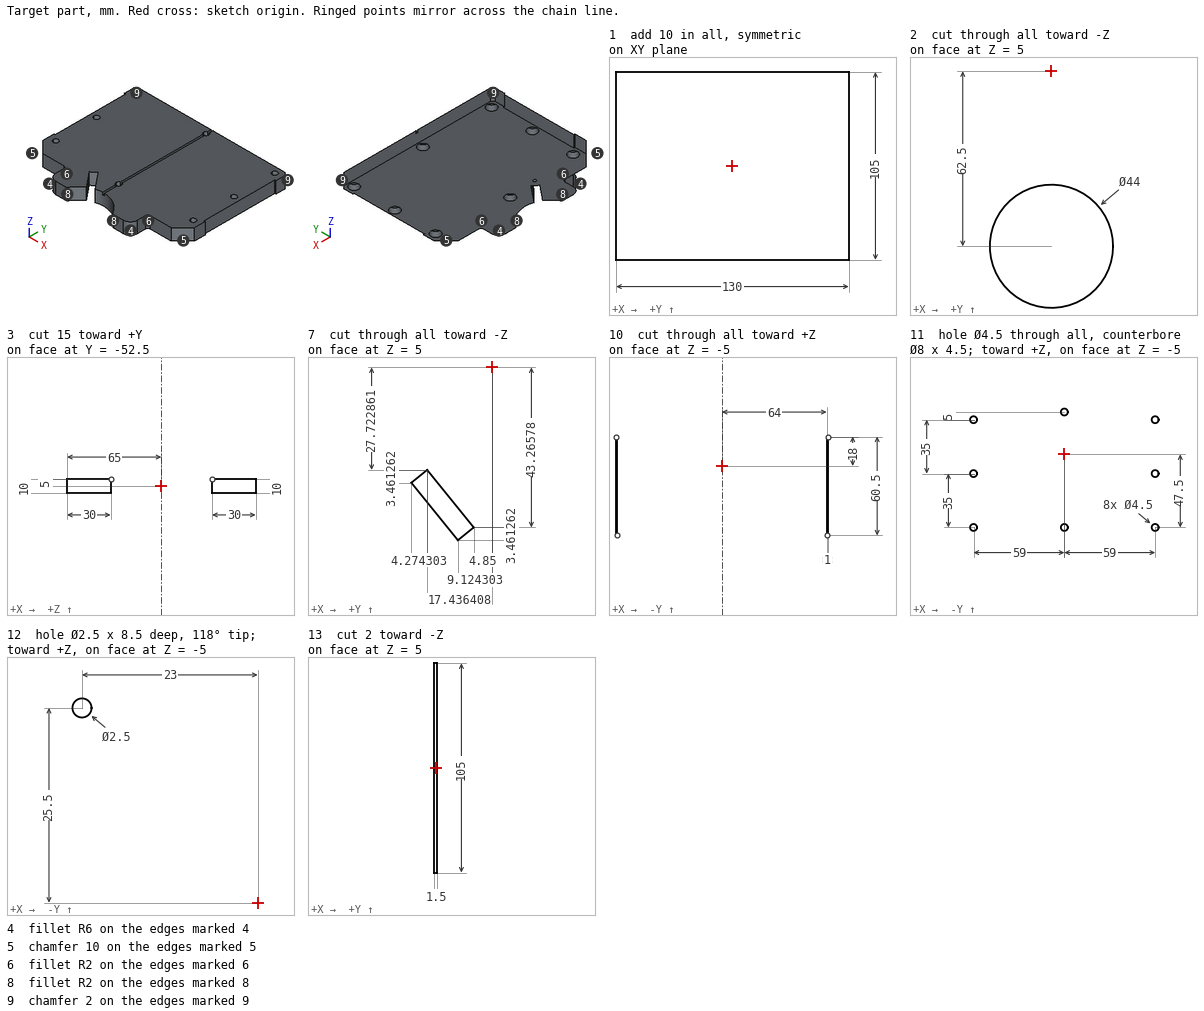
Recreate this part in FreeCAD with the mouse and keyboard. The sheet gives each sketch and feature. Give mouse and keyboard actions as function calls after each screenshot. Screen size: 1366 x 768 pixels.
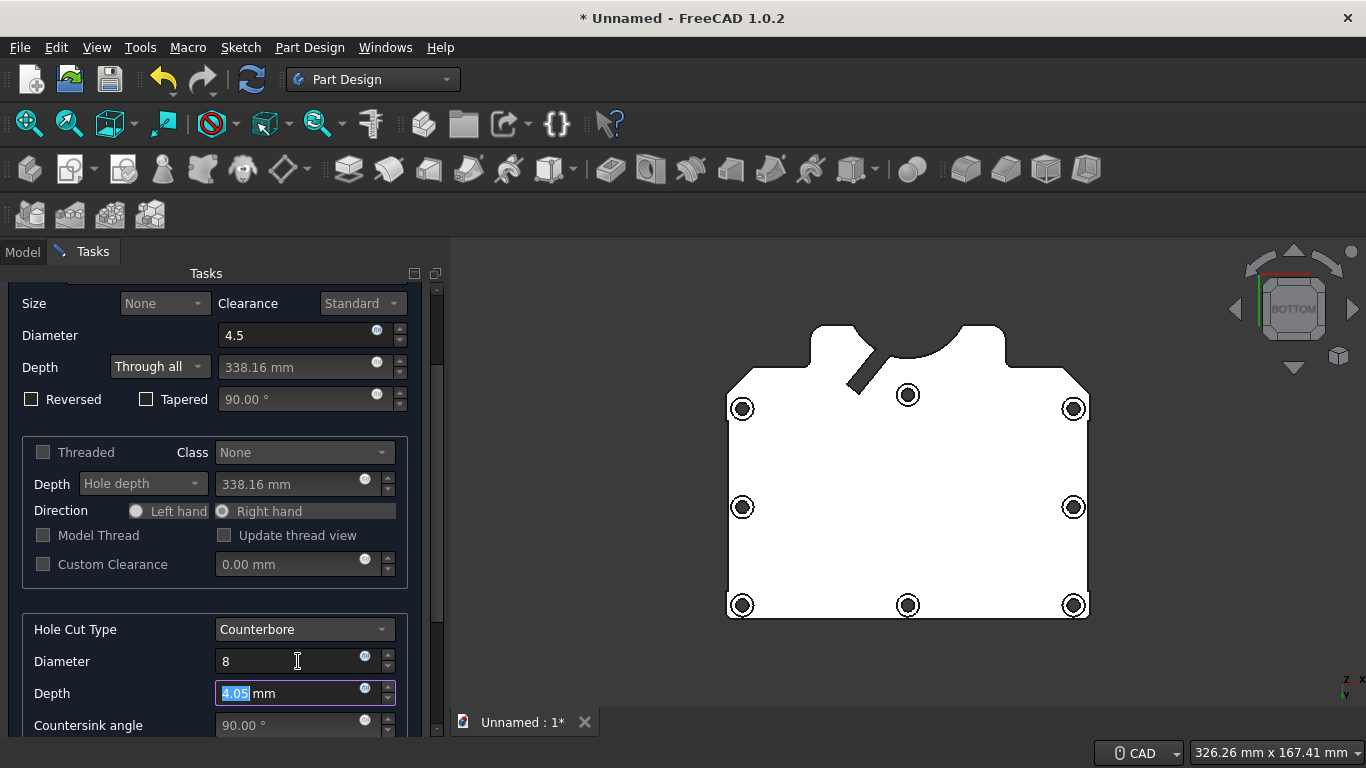
text(4.5)
key(Tab)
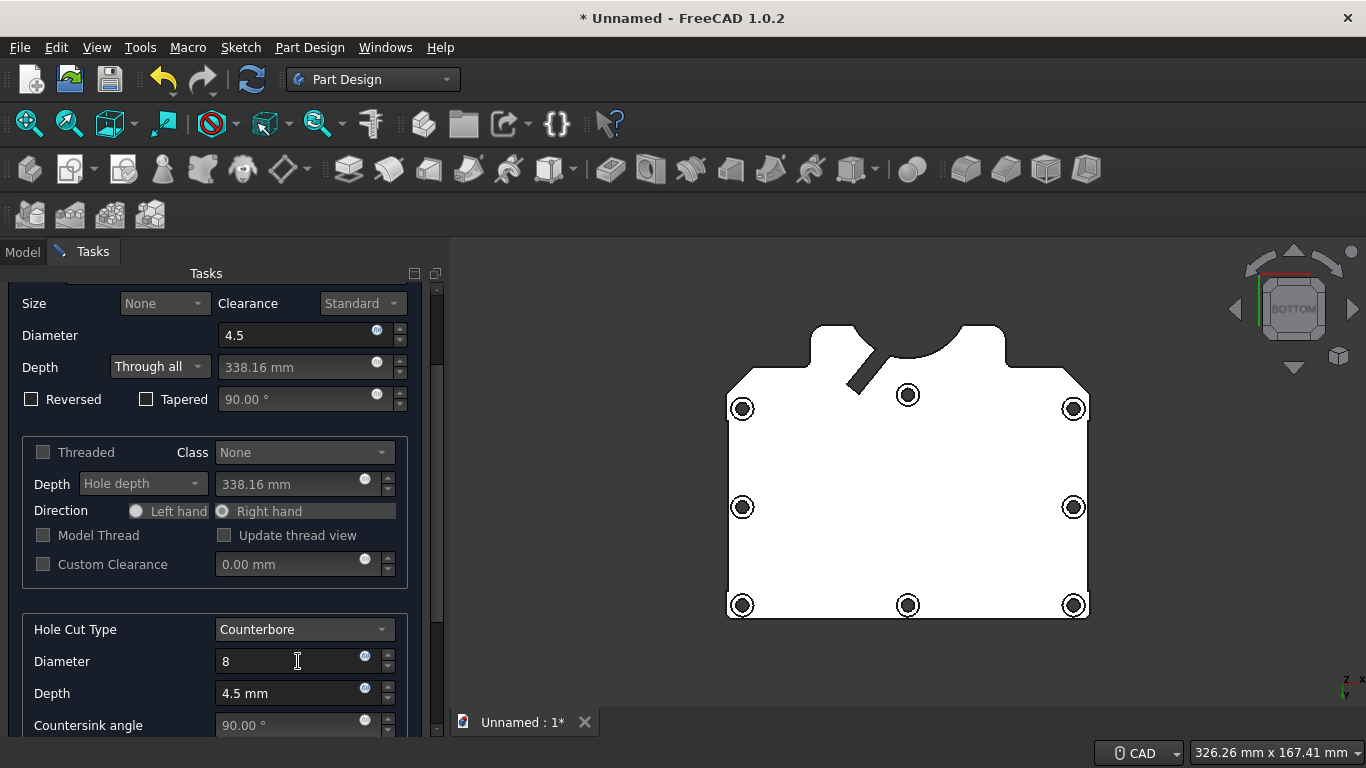
scroll(437, 510, up, 3)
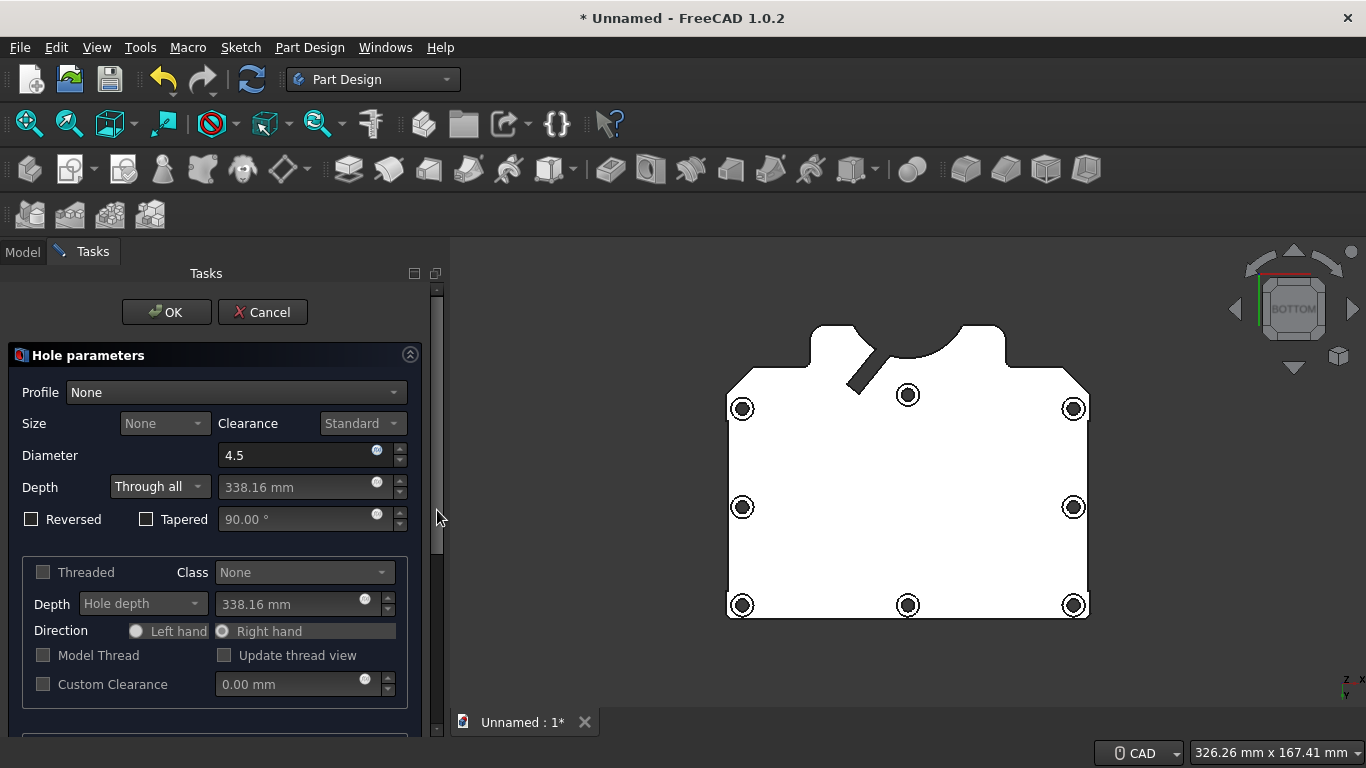
click(167, 312)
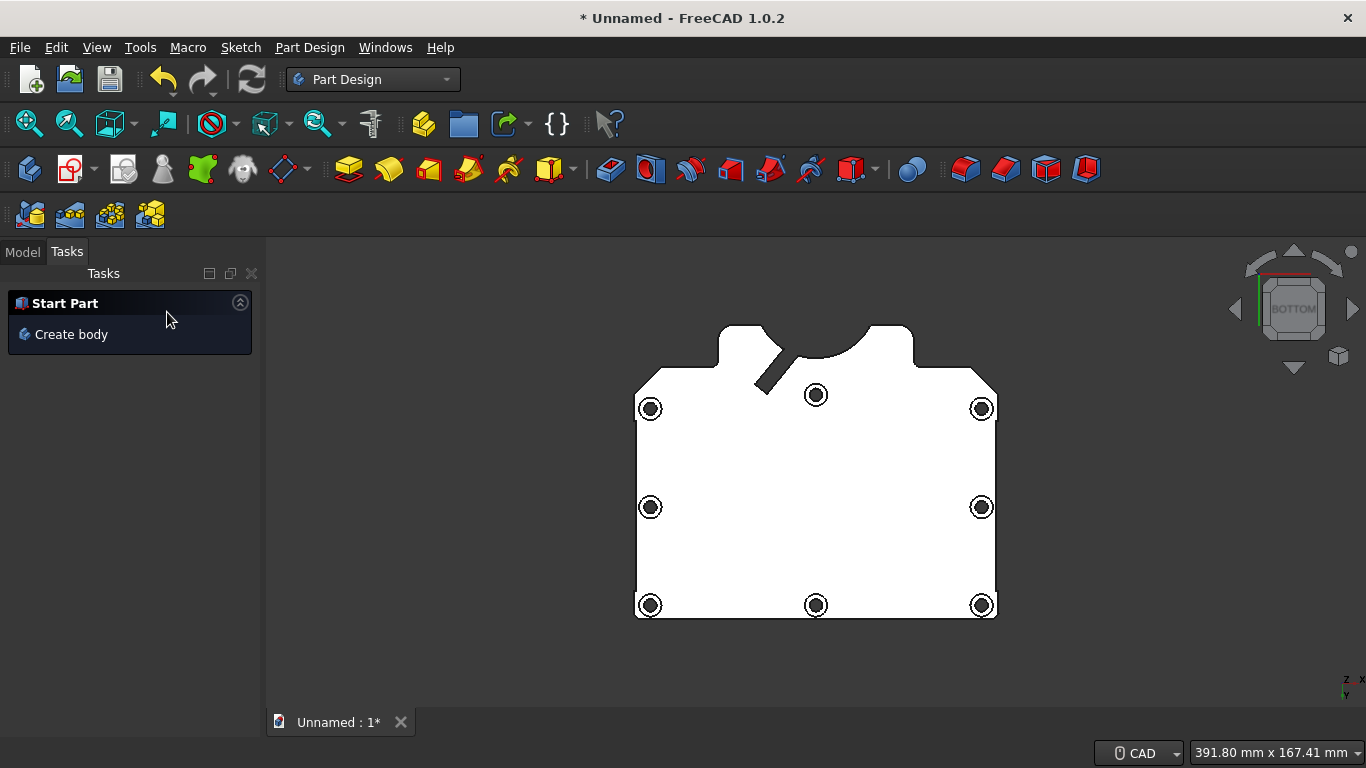
click(868, 513)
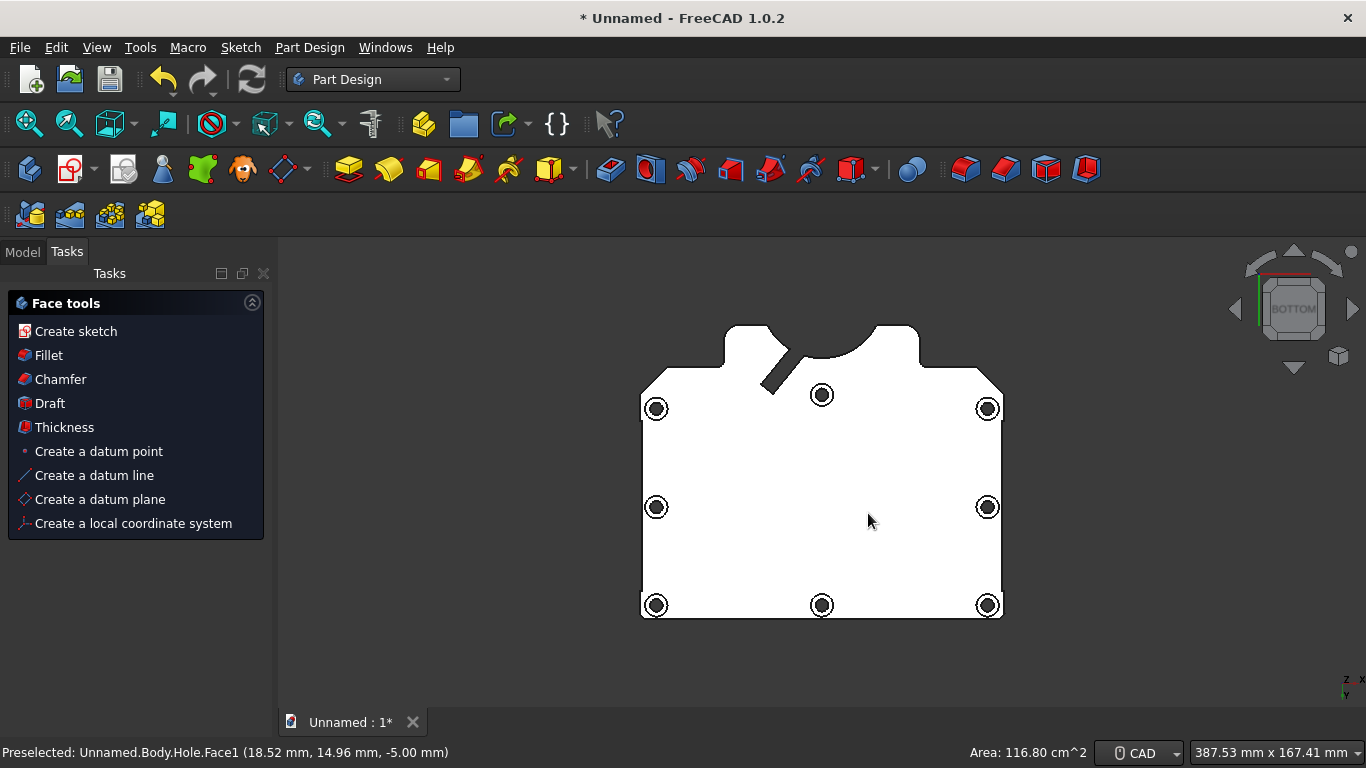
click(70, 170)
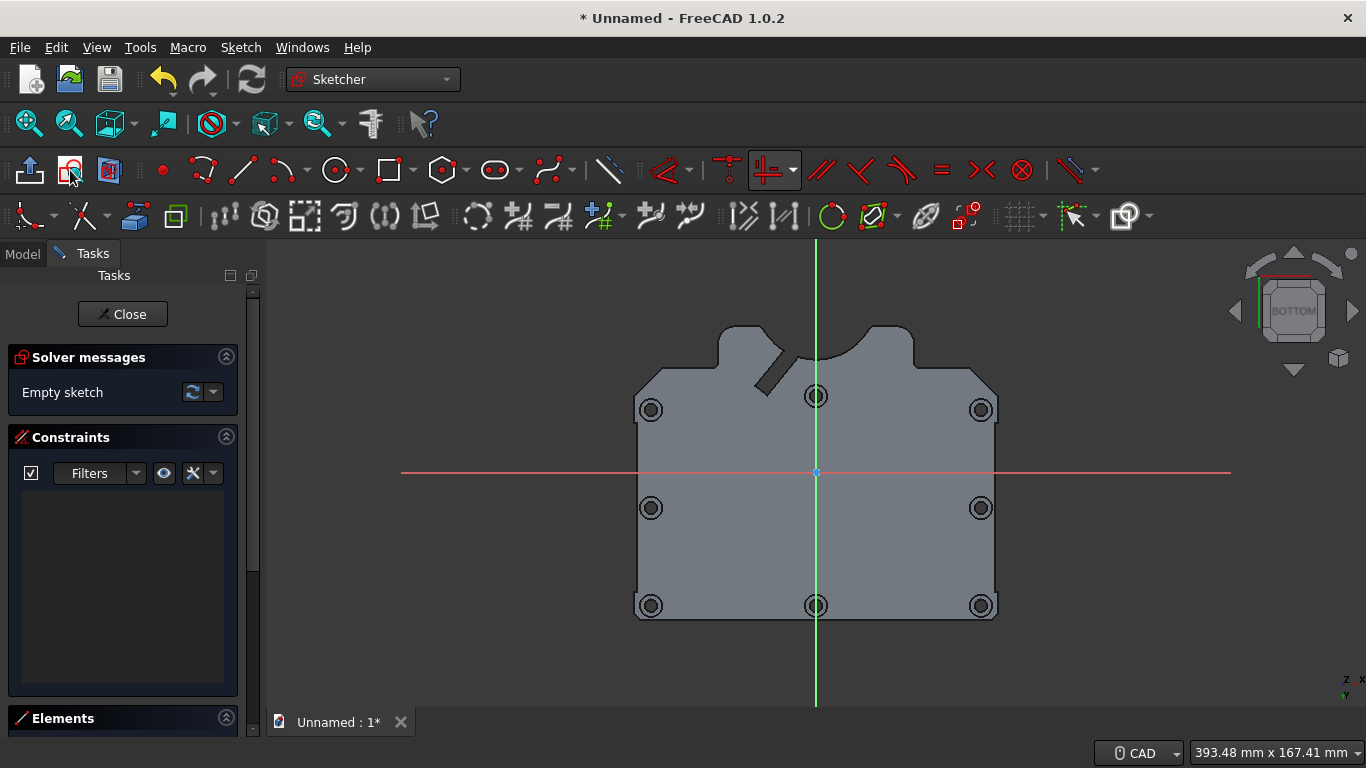
scroll(752, 398, up, 15)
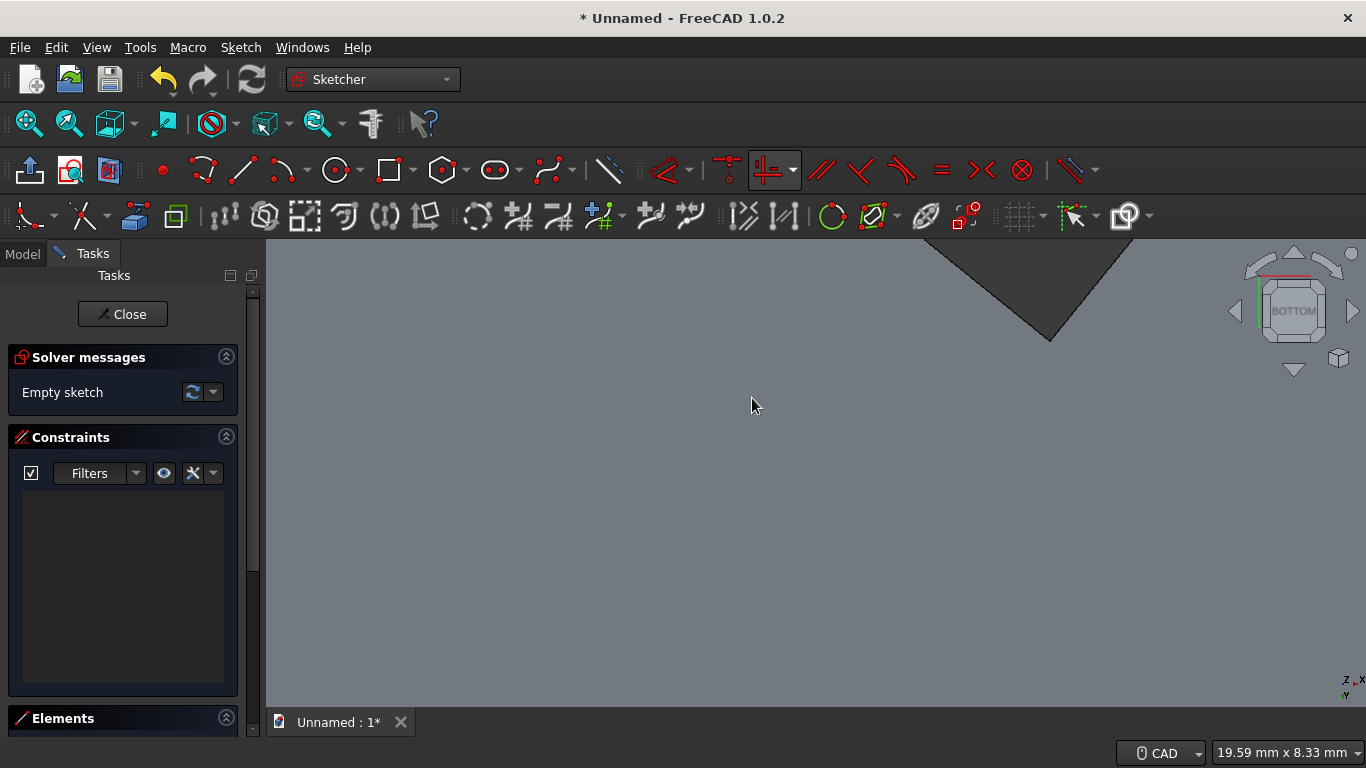
scroll(729, 460, up, 4)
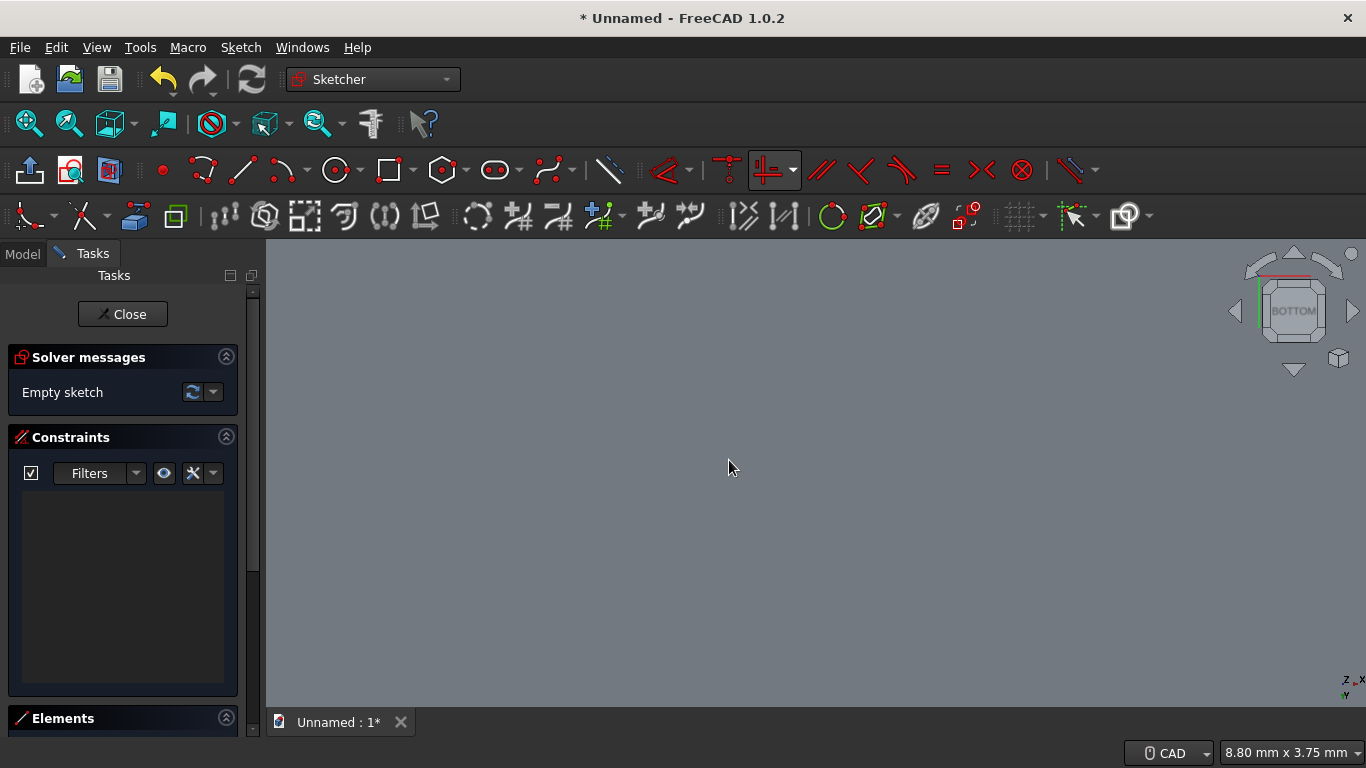
click(336, 170)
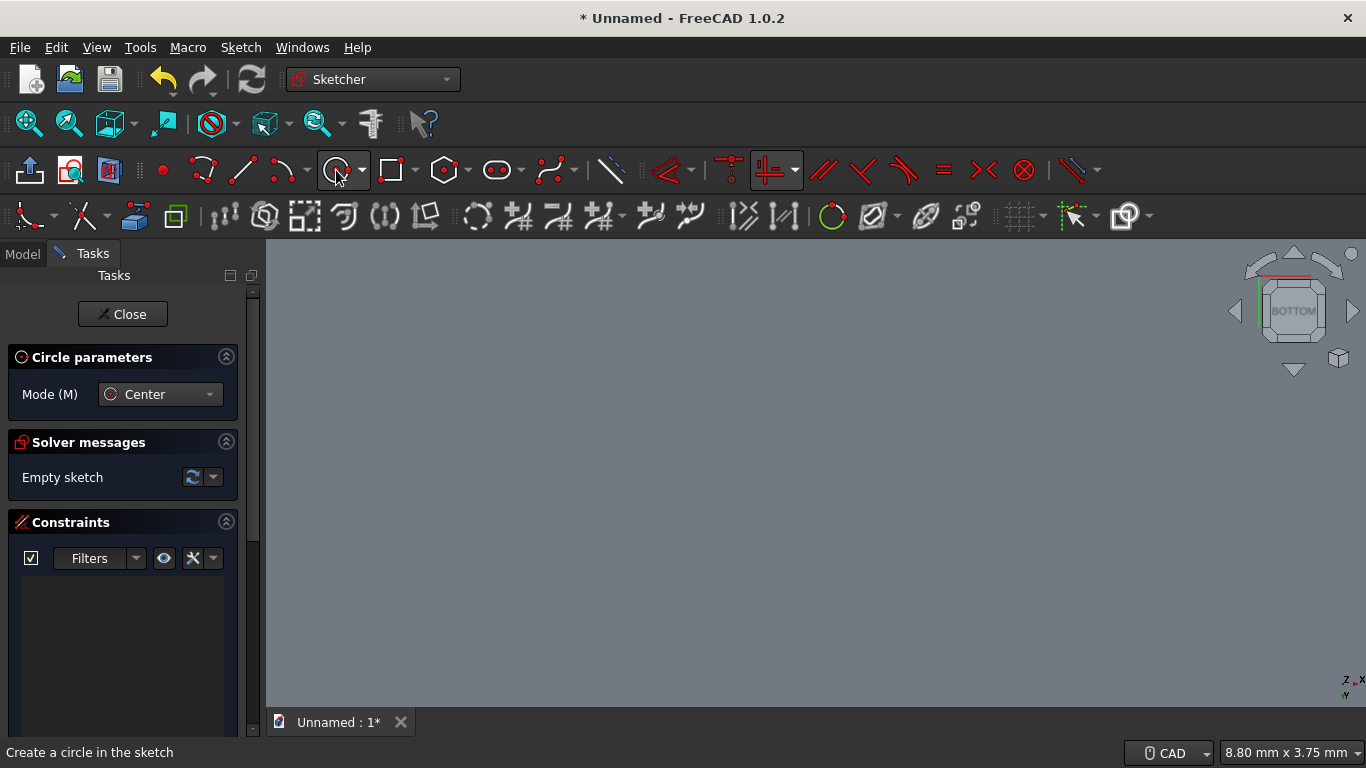
click(748, 473)
move(858, 362)